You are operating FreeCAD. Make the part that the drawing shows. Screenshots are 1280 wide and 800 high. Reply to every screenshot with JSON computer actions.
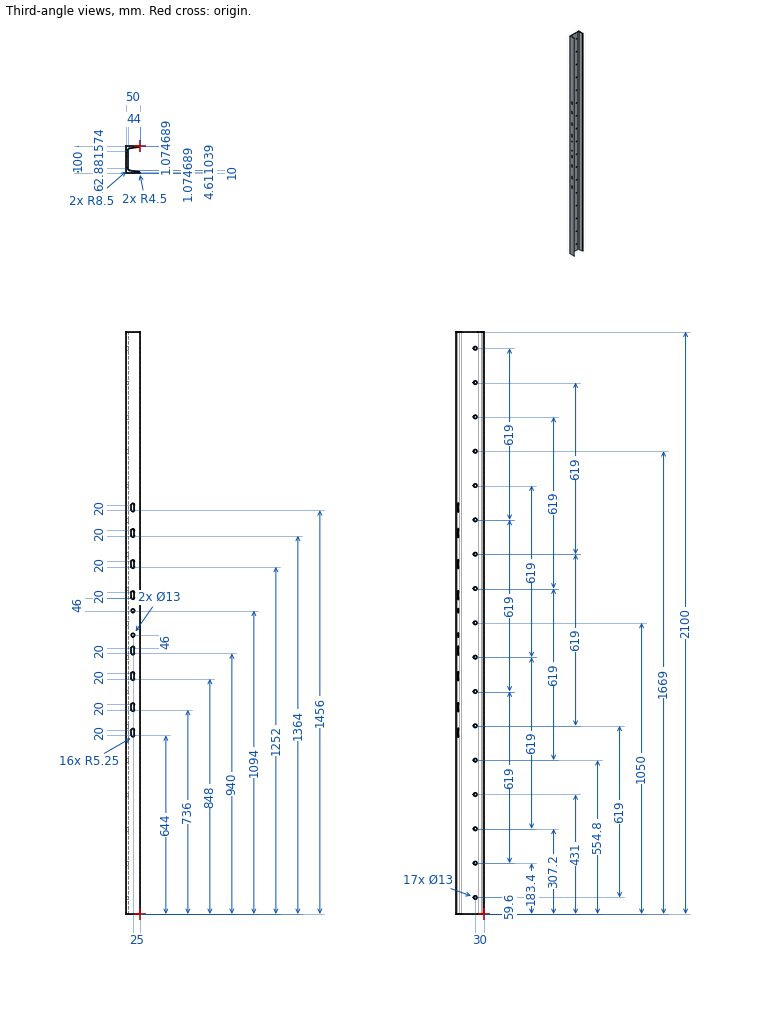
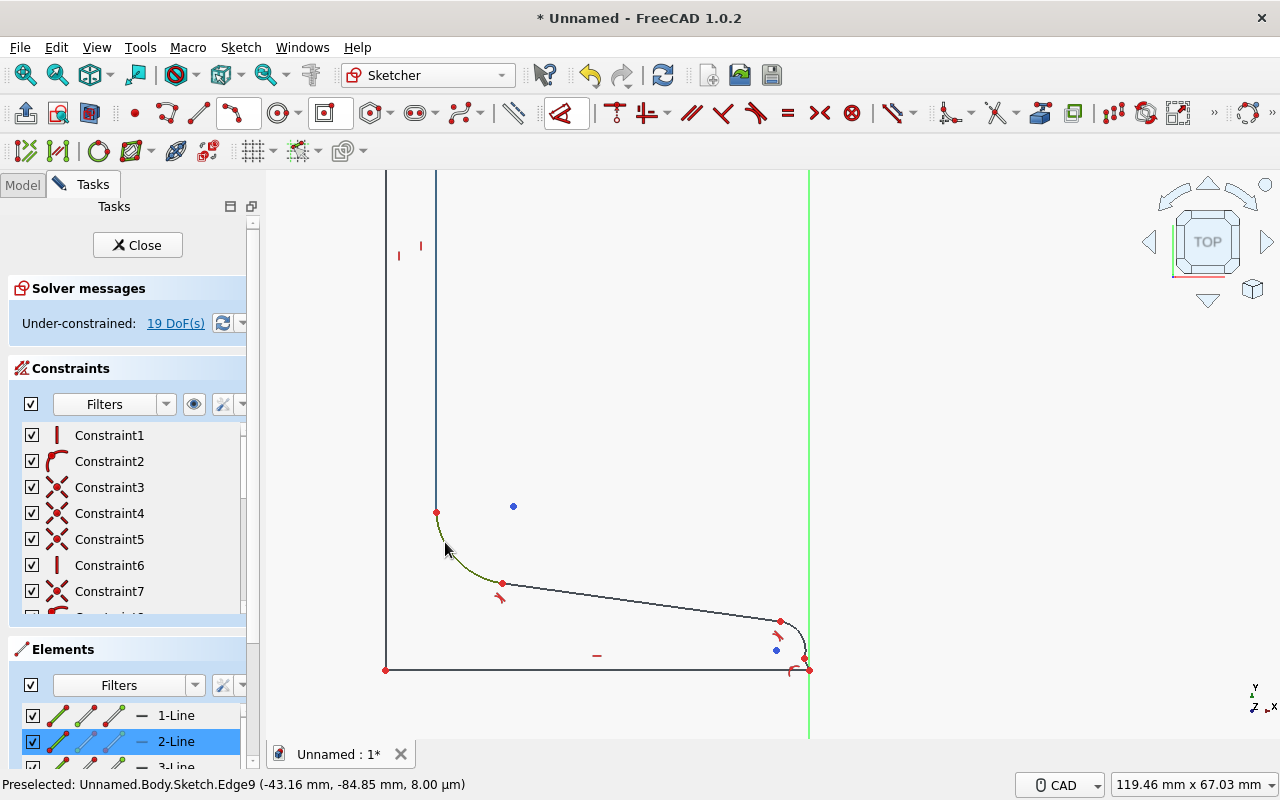
{"action": "key", "text": "t"}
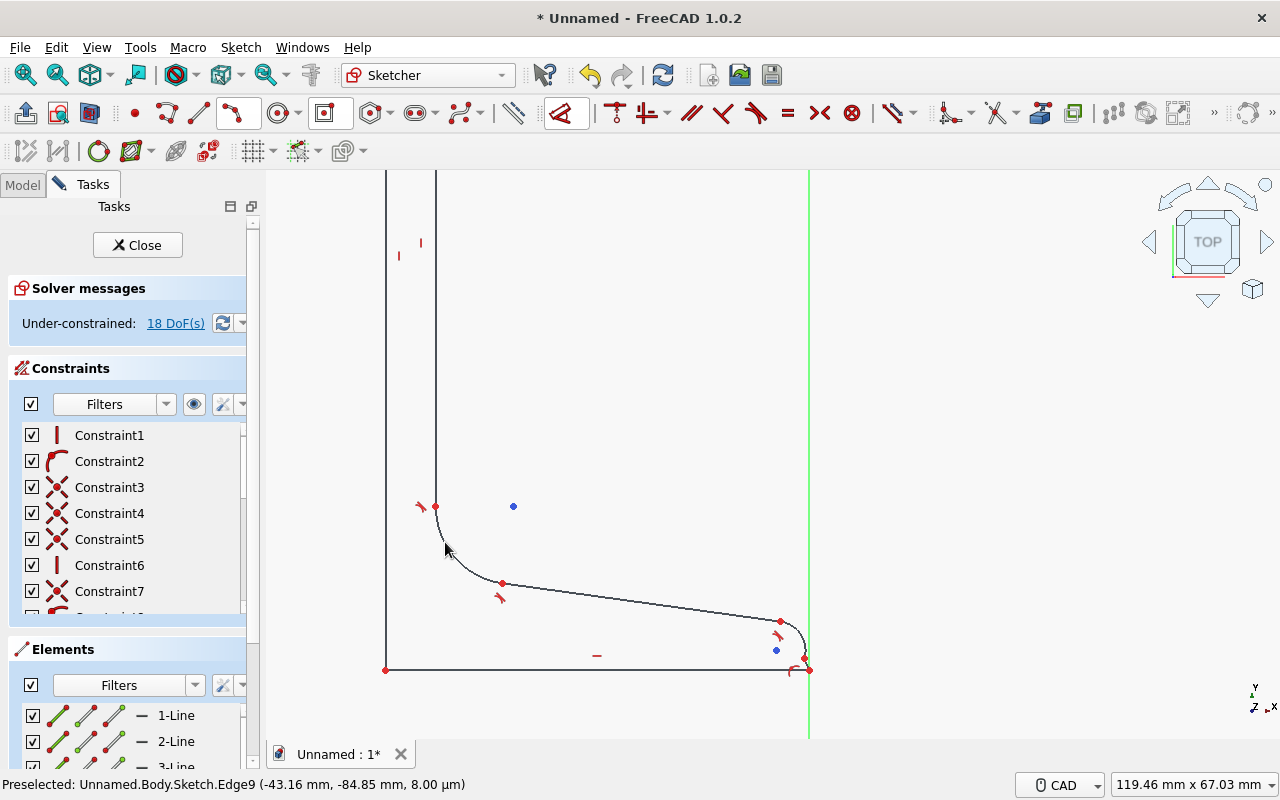
{"action": "left_click", "coordinate": [436, 348]}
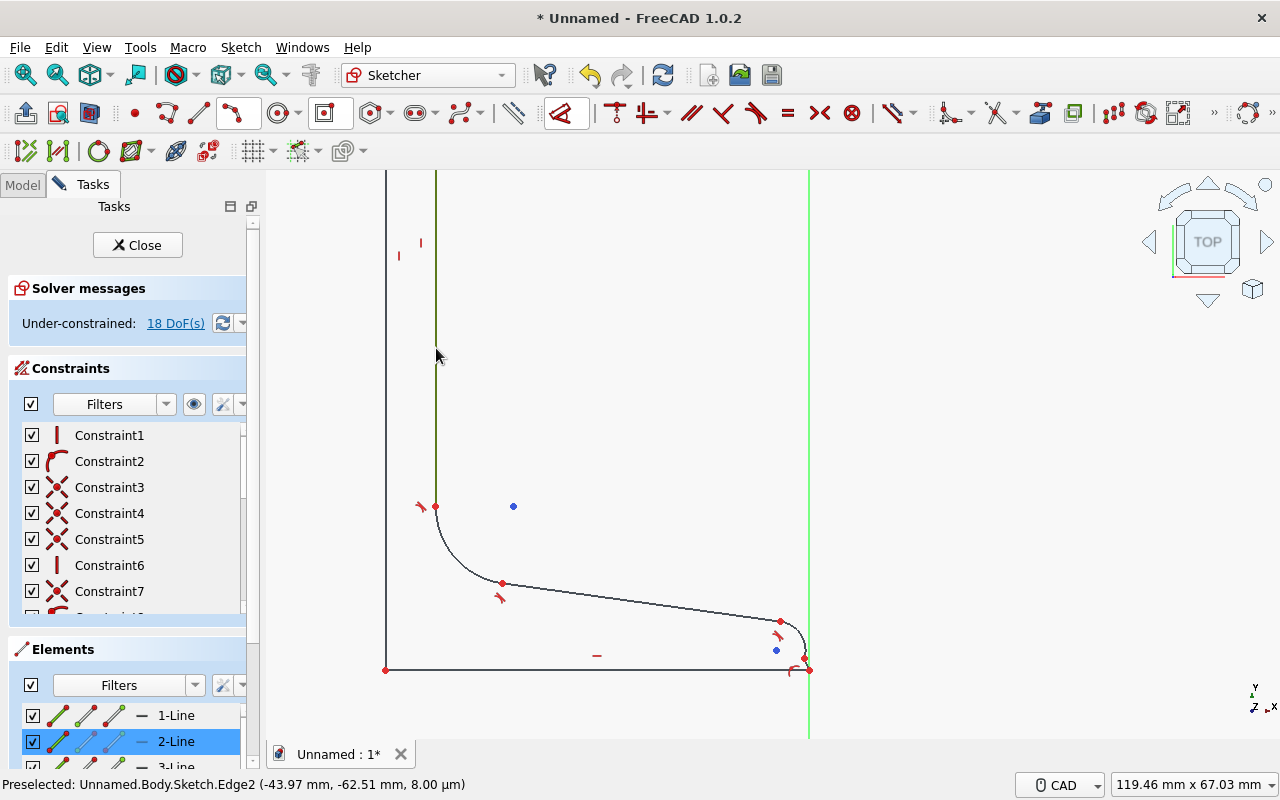
{"action": "scroll", "coordinate": [792, 627], "scroll_direction": "down", "scroll_amount": 4}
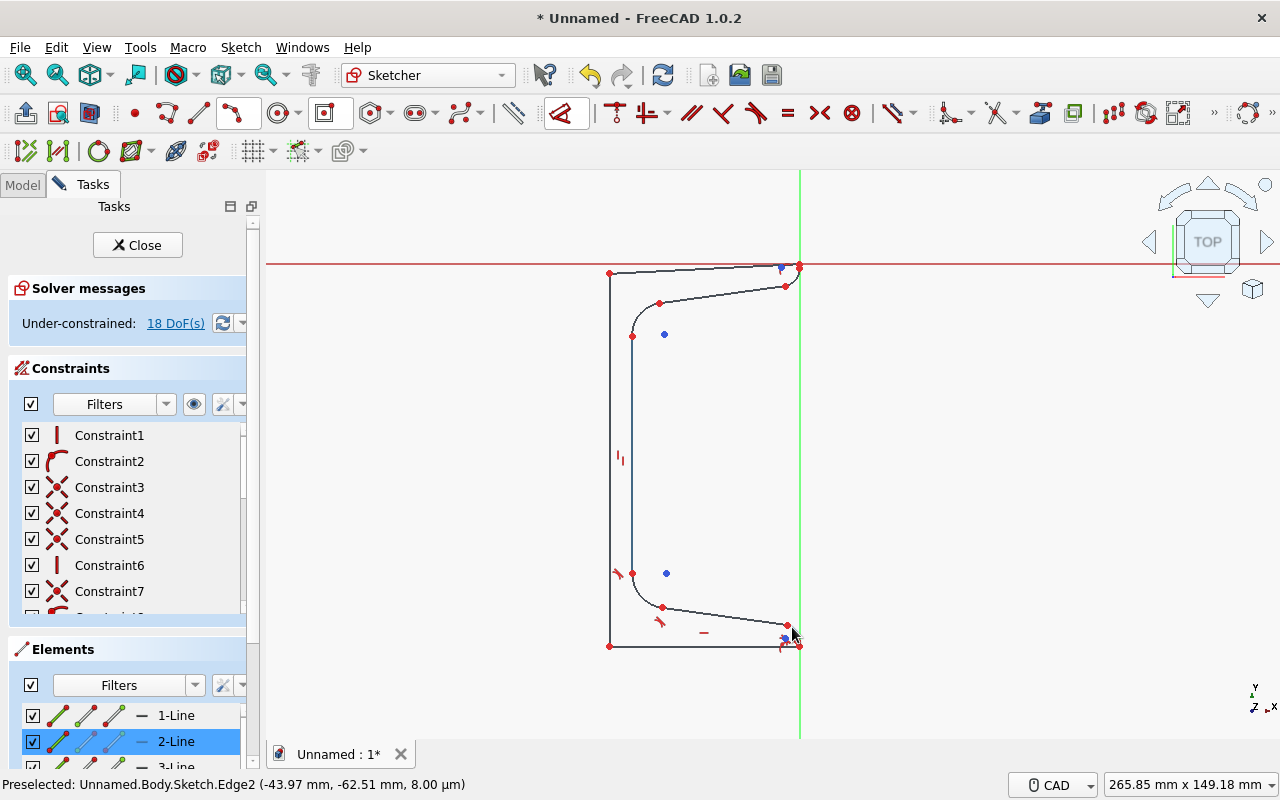
{"action": "left_click", "coordinate": [647, 308]}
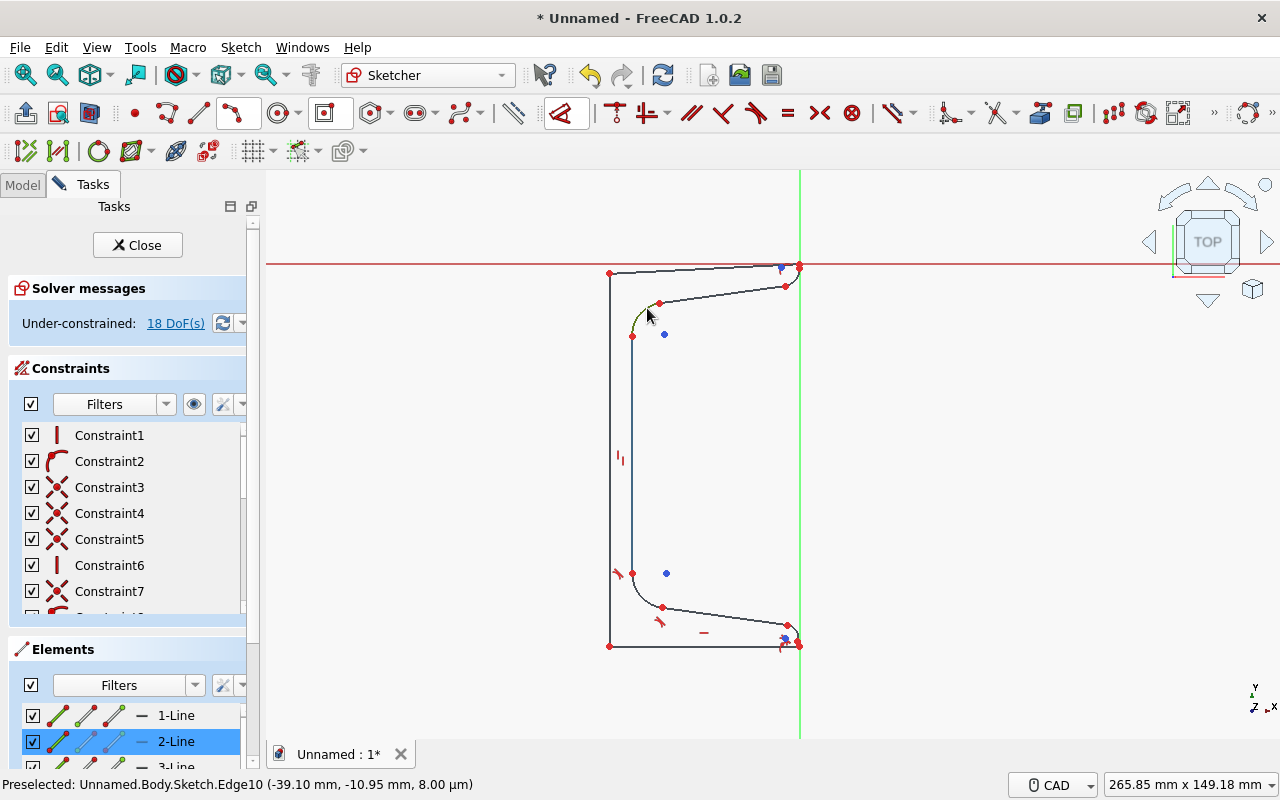
{"action": "left_click", "coordinate": [756, 114]}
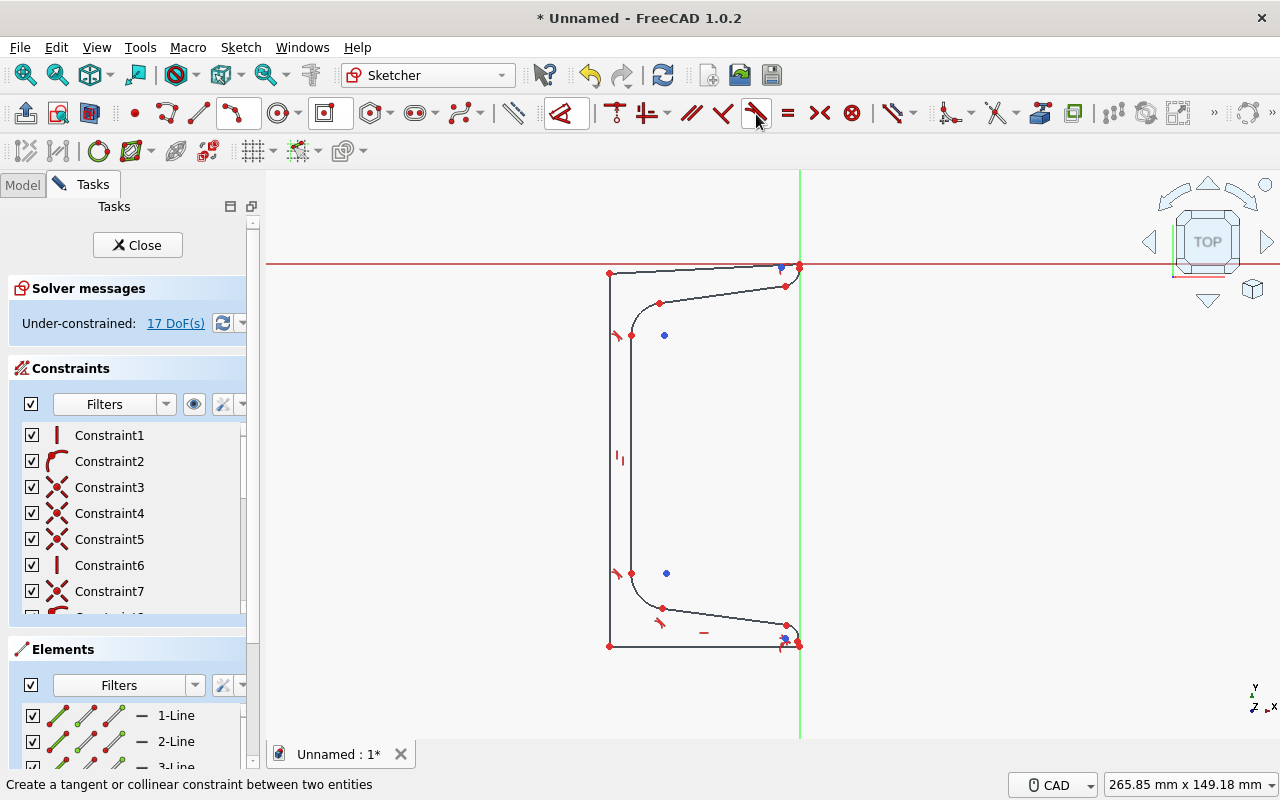
{"action": "left_click", "coordinate": [697, 298]}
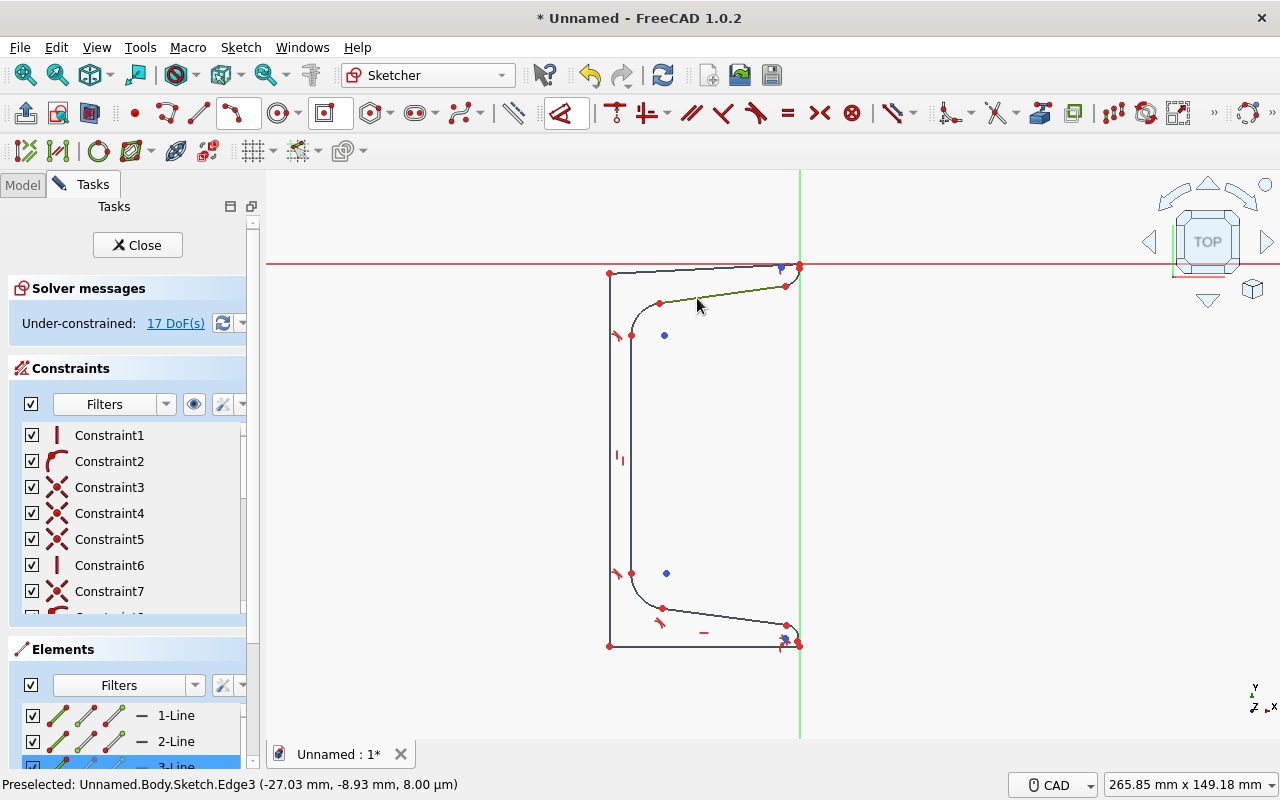
{"action": "left_click", "coordinate": [647, 308]}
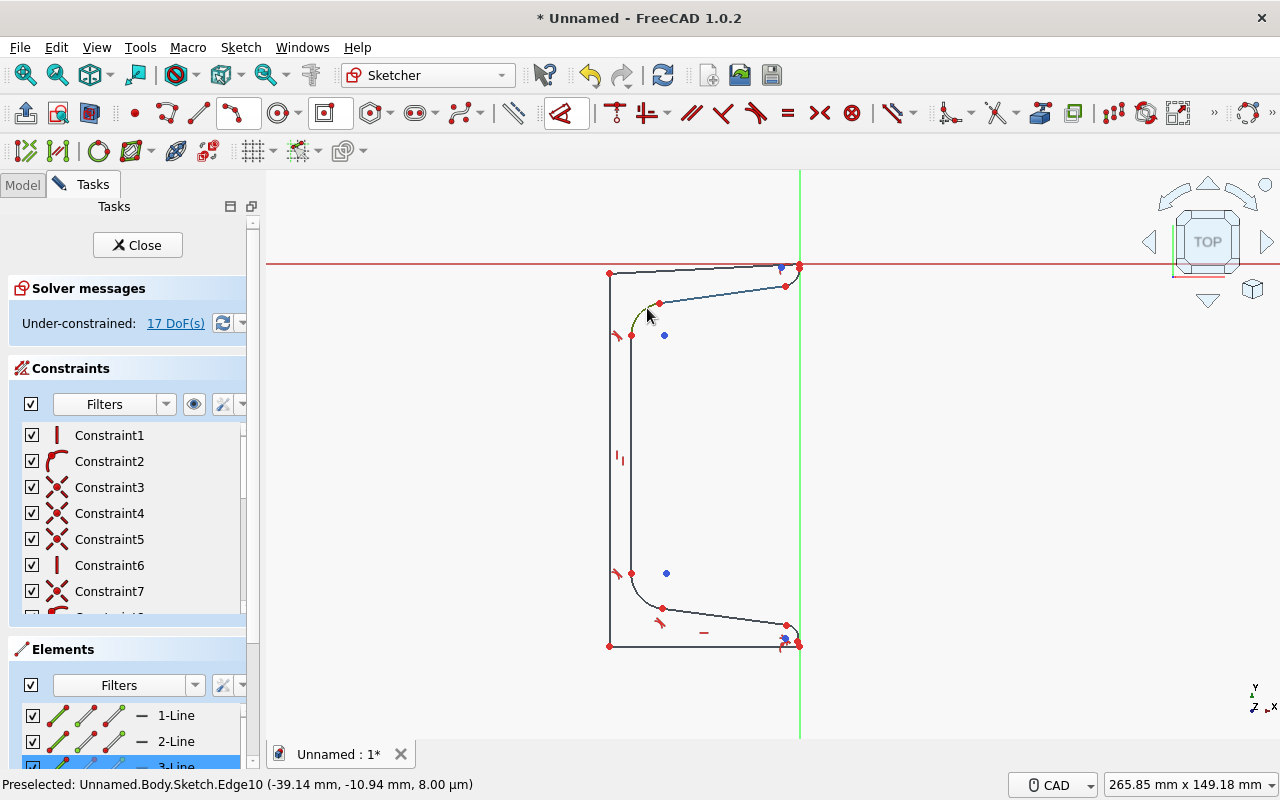
{"action": "key", "text": "t"}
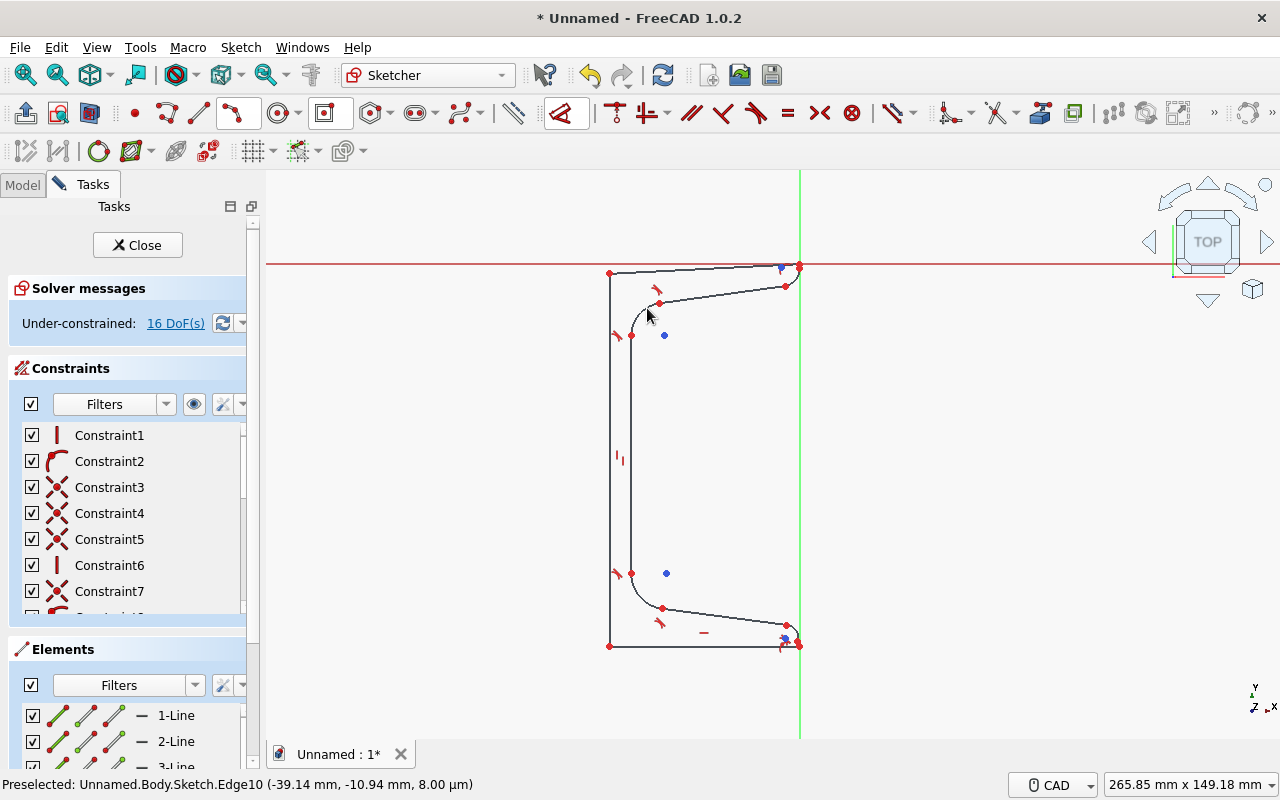
{"action": "left_click", "coordinate": [697, 298]}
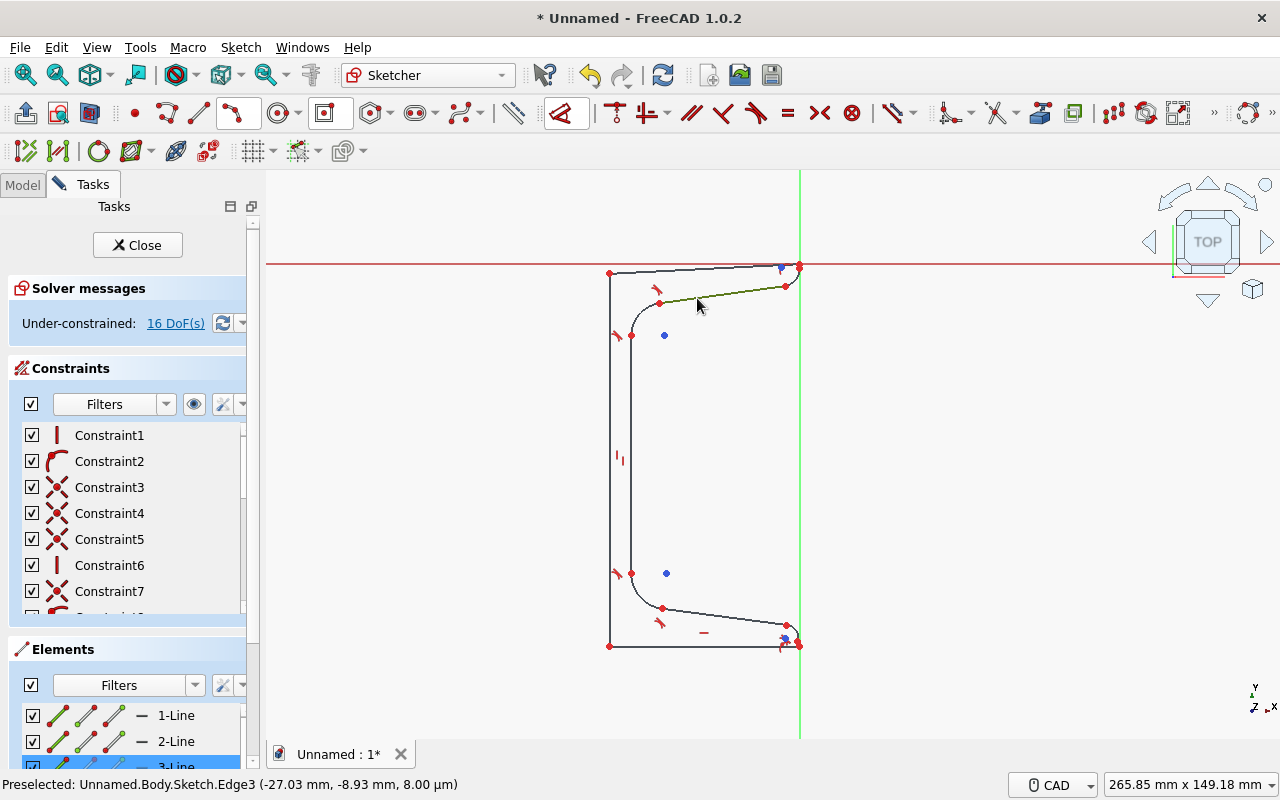
{"action": "scroll", "coordinate": [798, 276], "scroll_direction": "up", "scroll_amount": 4}